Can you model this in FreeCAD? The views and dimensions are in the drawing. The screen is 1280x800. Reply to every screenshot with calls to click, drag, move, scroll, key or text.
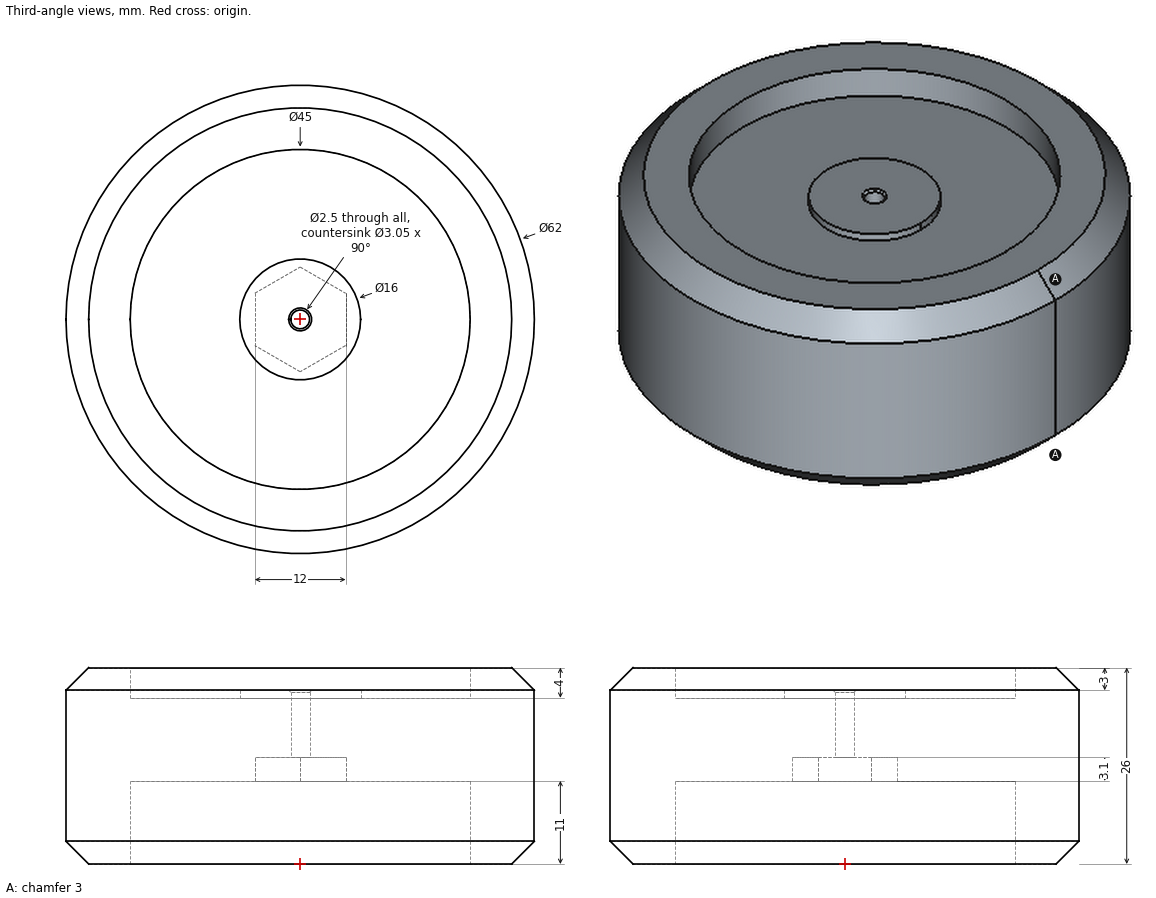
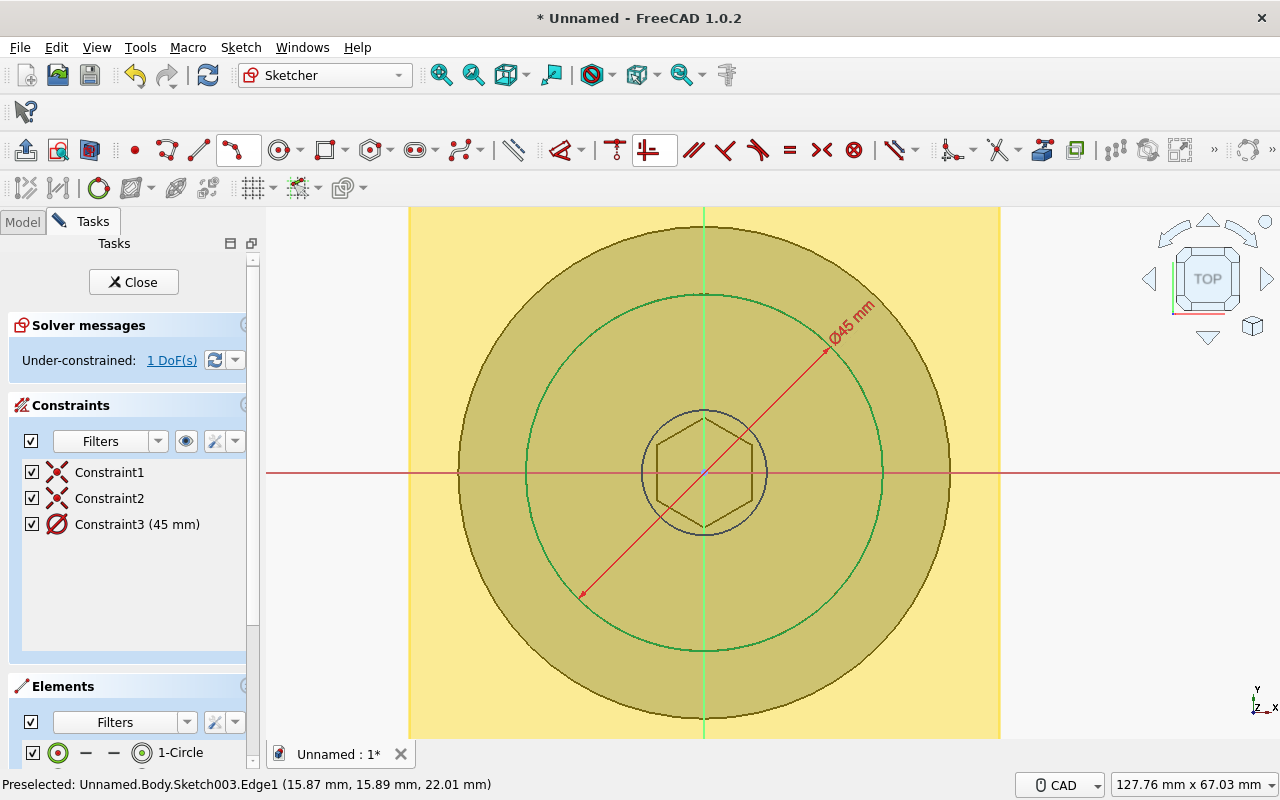
click(748, 428)
click(770, 405)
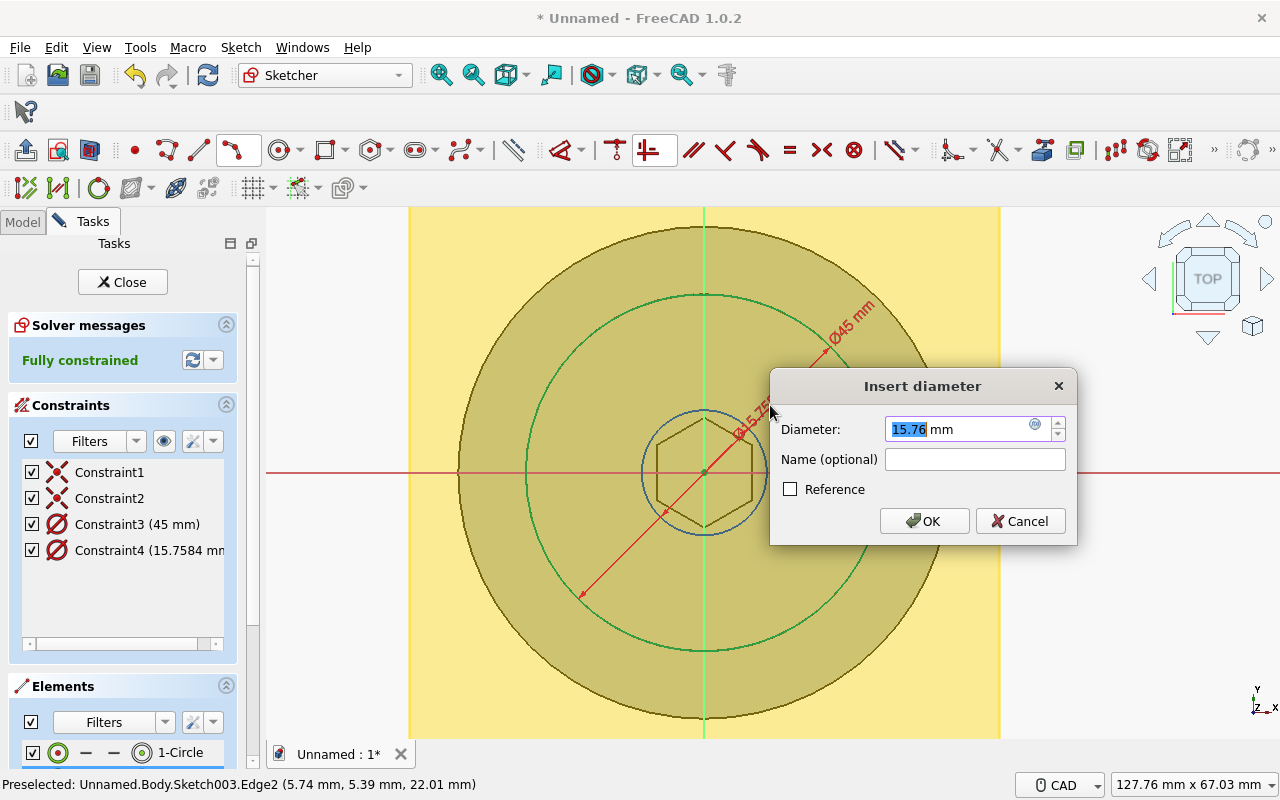
text(16)
key(Return)
key(Escape)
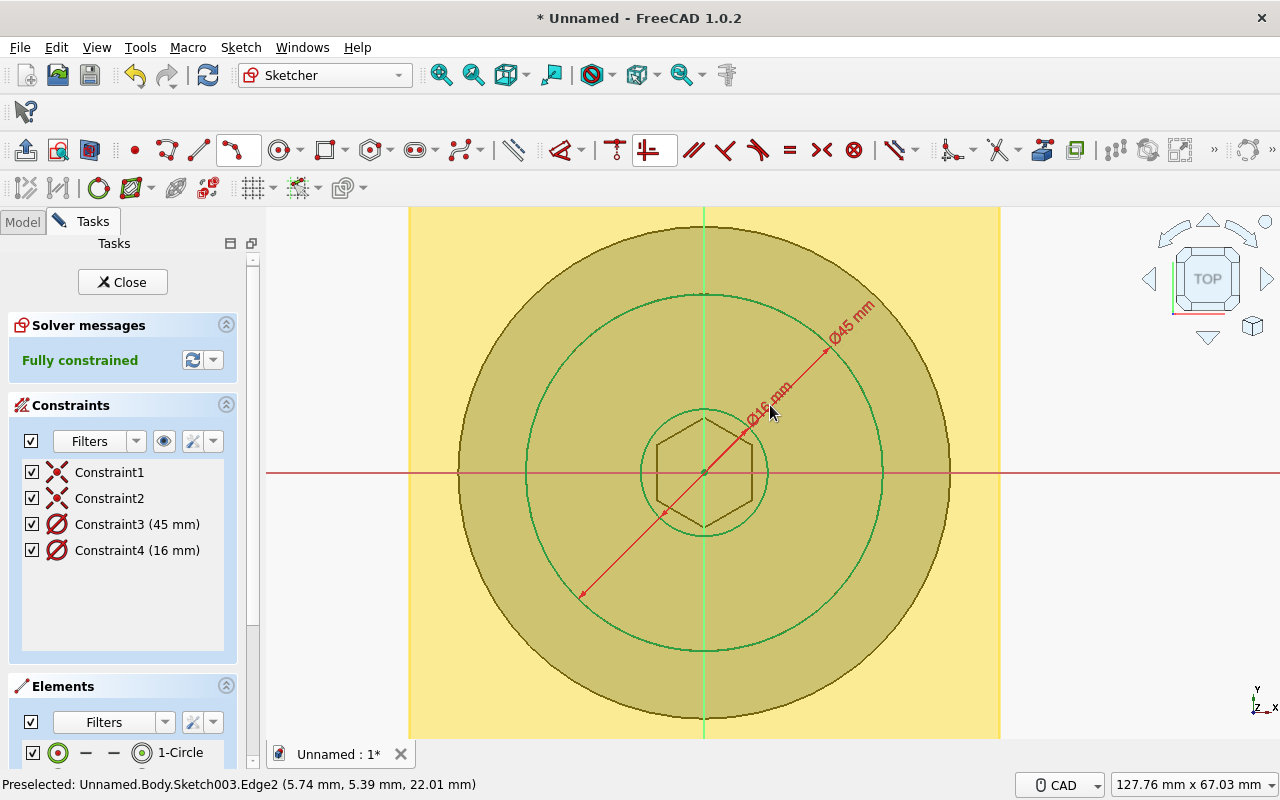
click(123, 282)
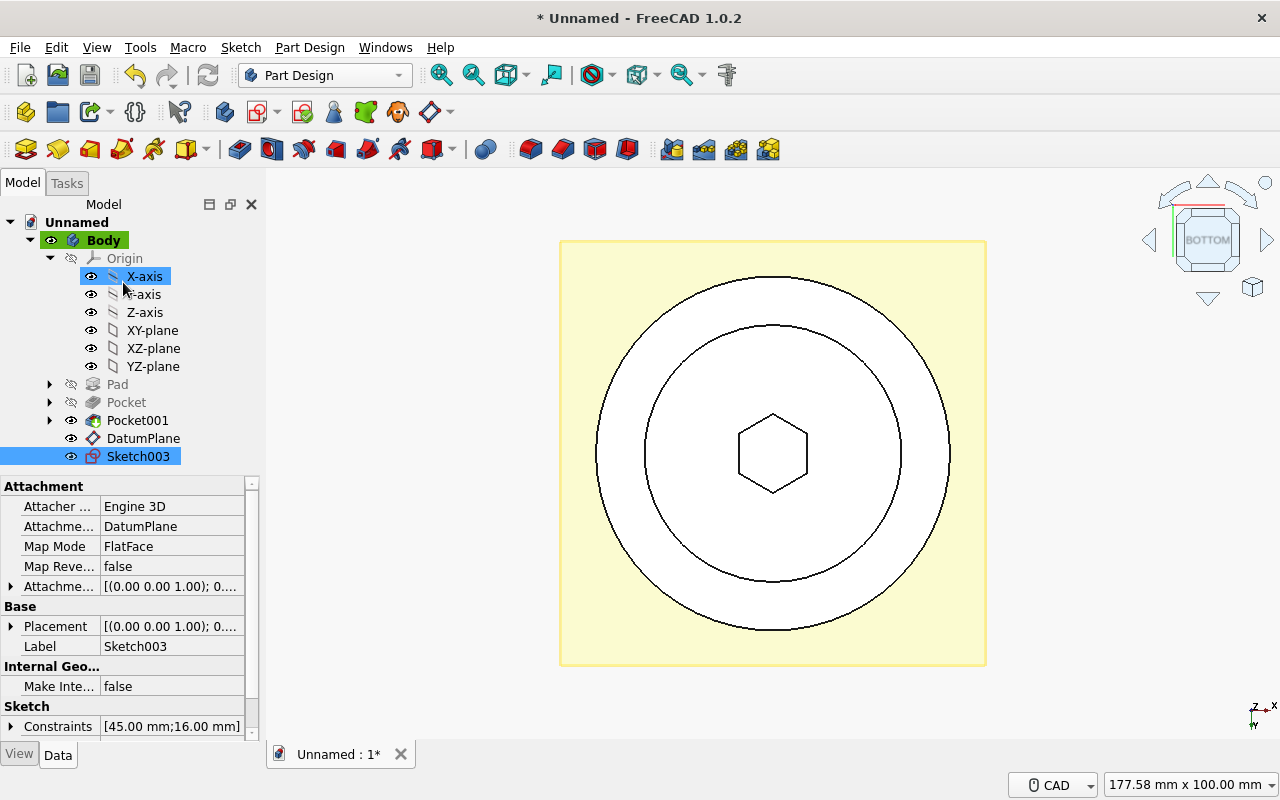
click(240, 150)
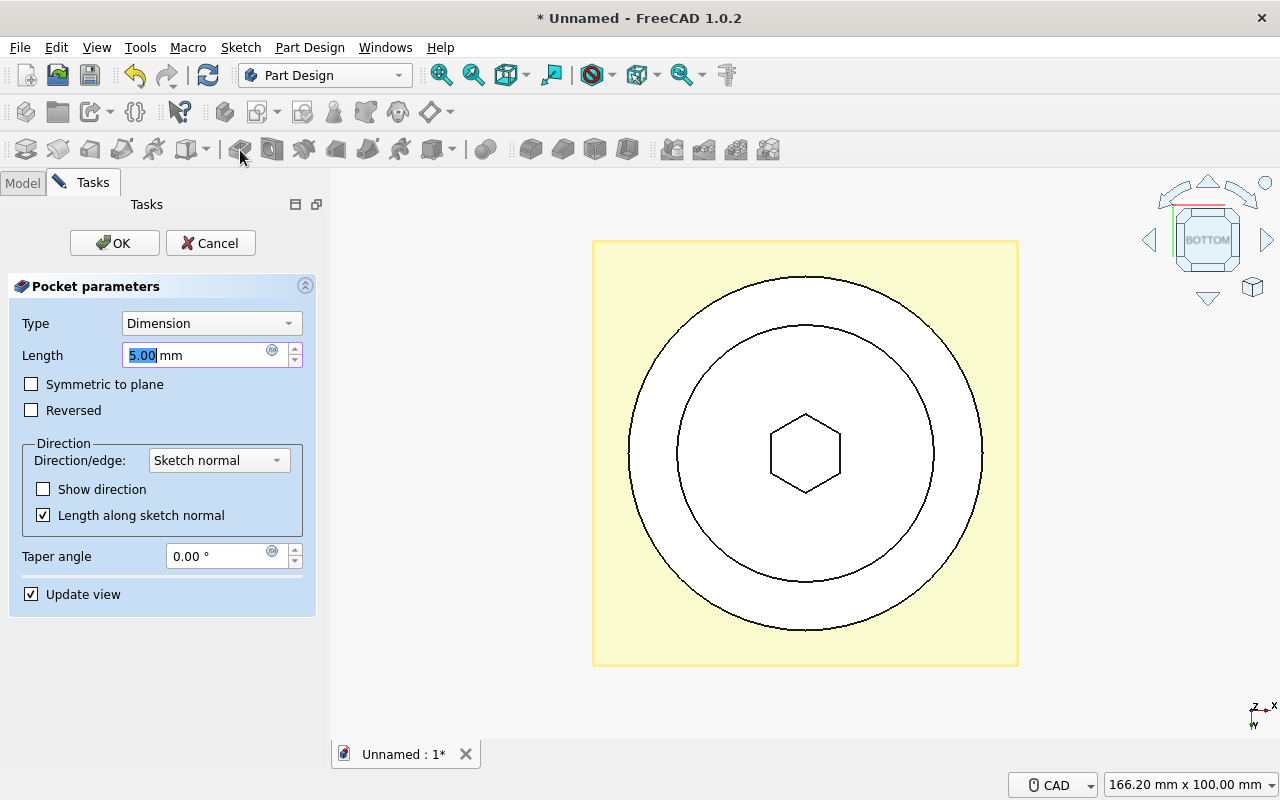
text(4)
key(Tab)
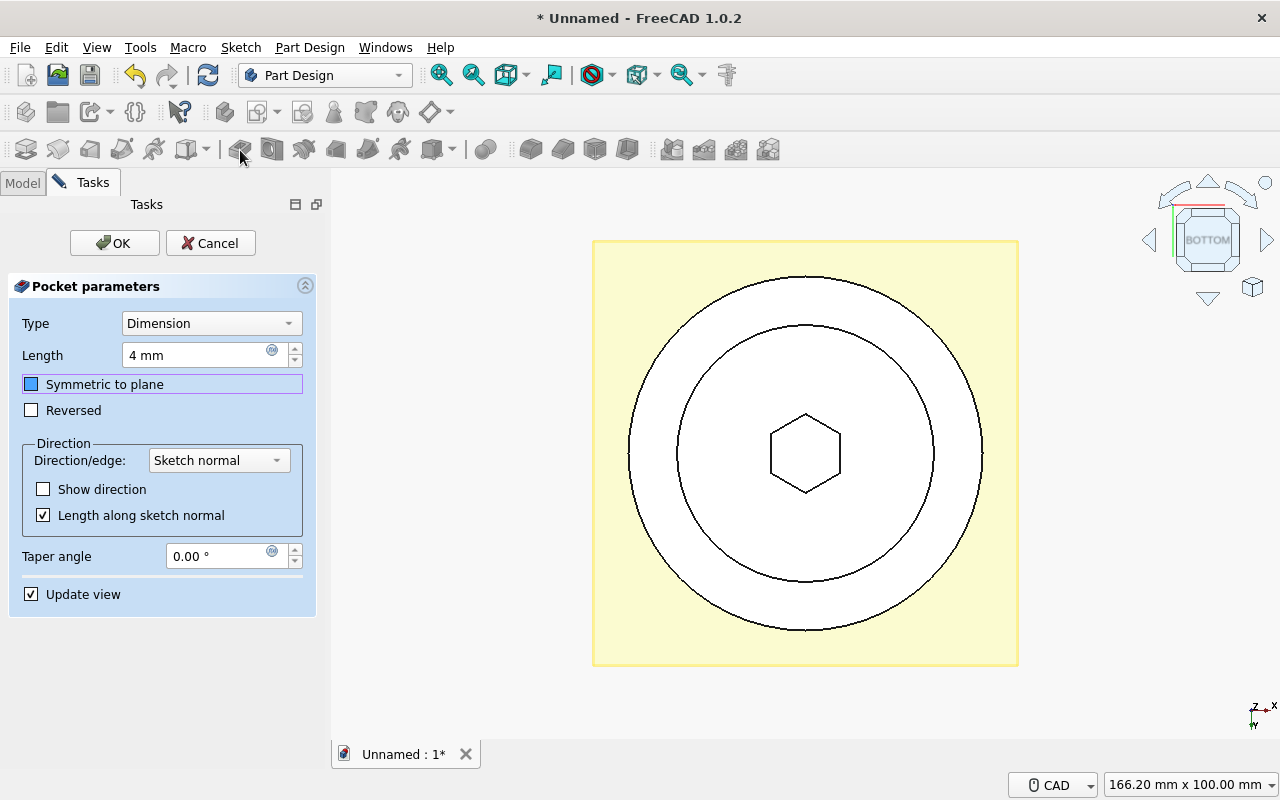
click(30, 410)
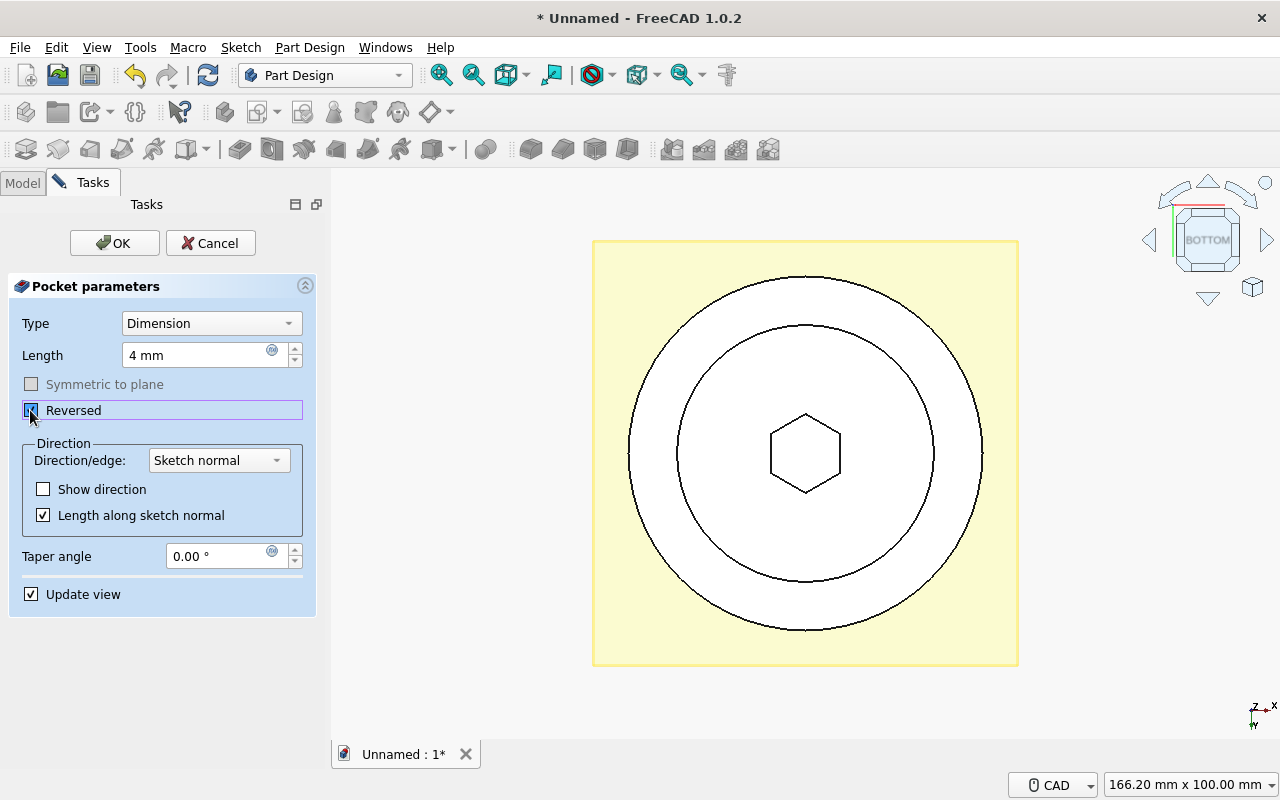
click(115, 243)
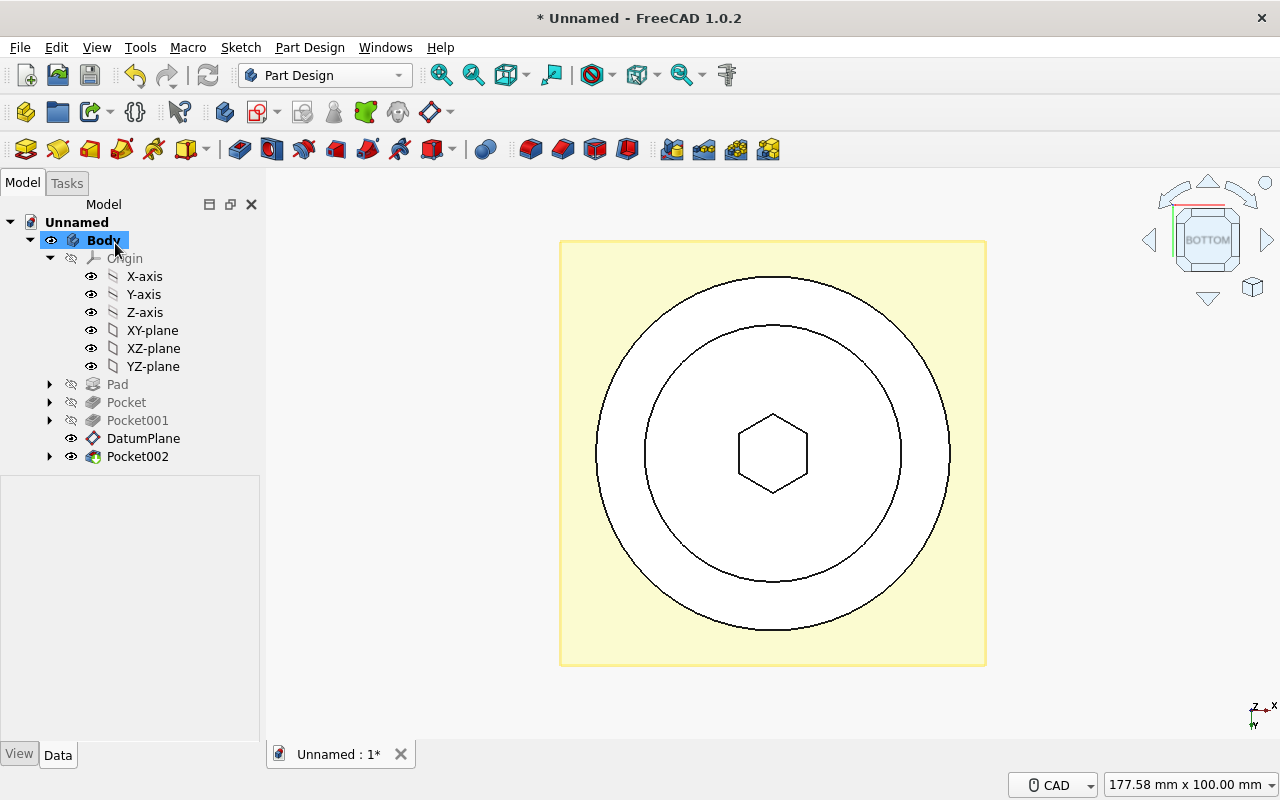
click(116, 438)
key(space)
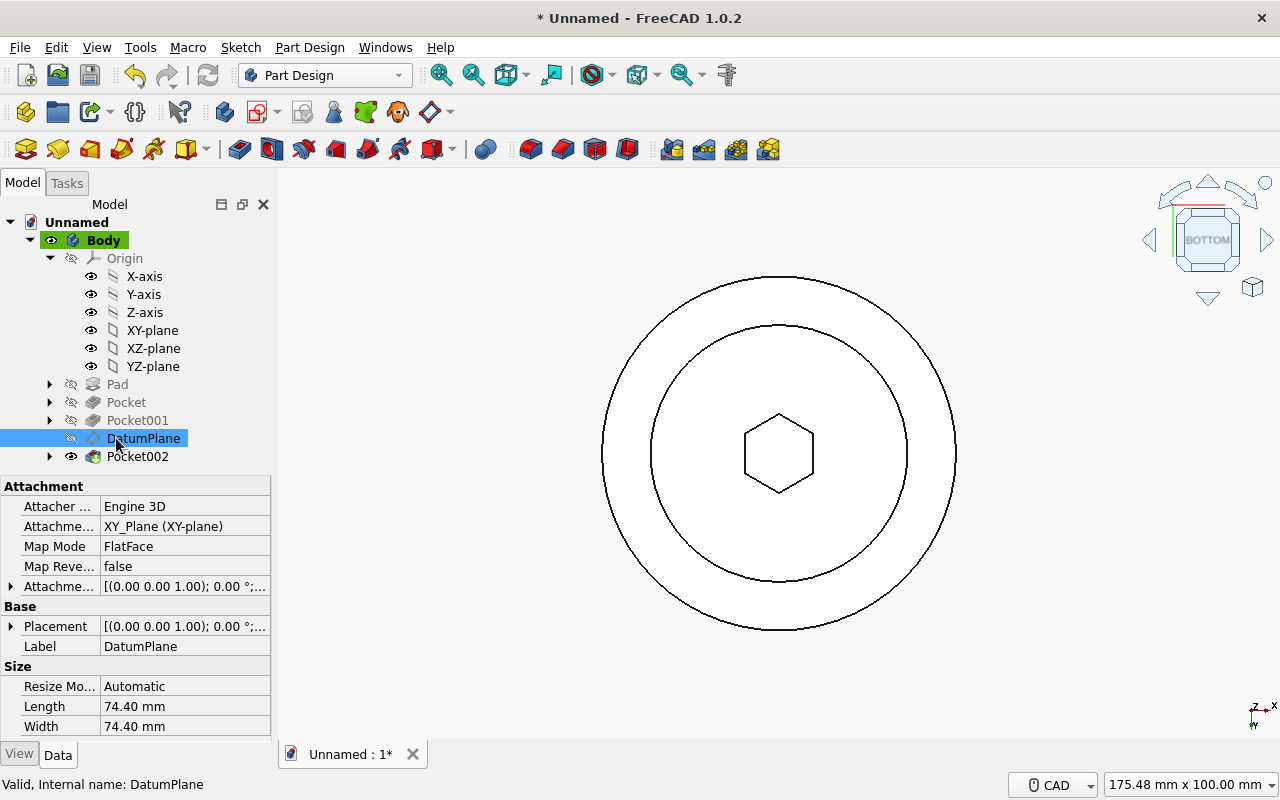
click(136, 330)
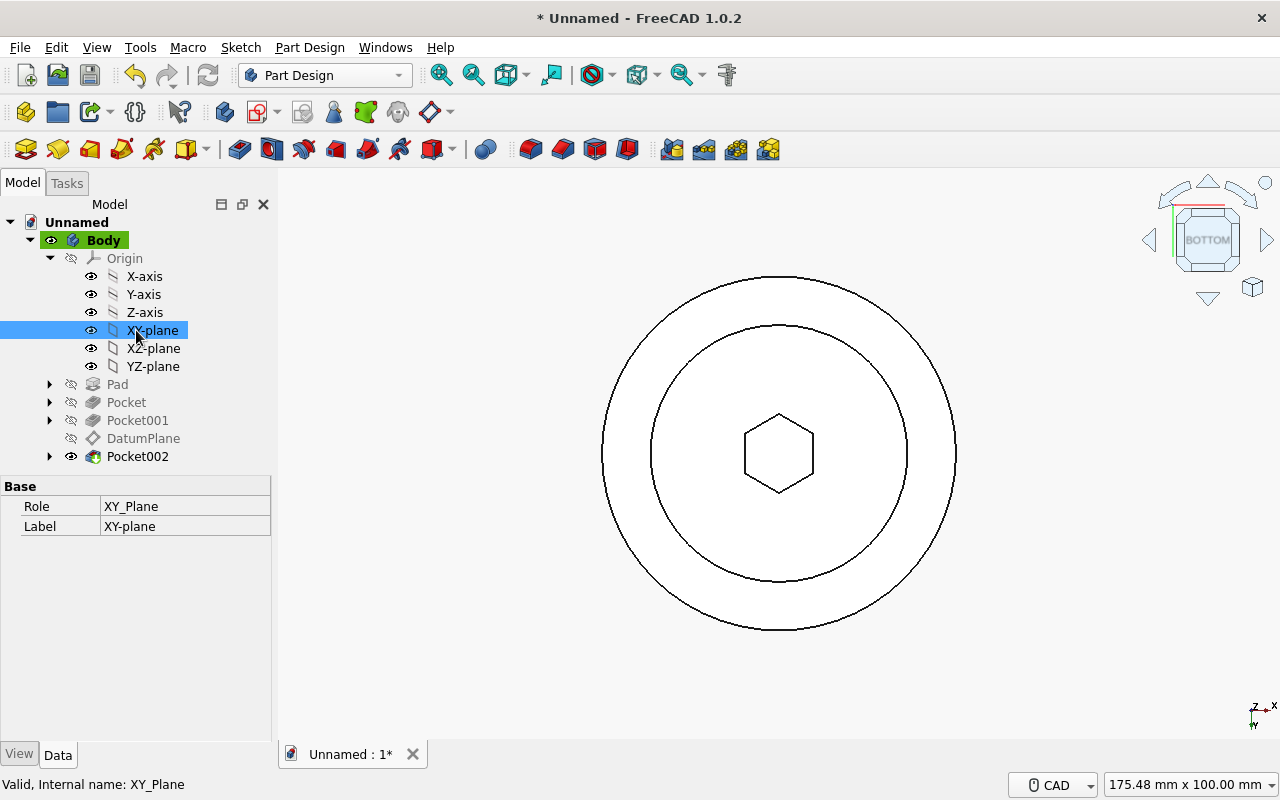
click(430, 112)